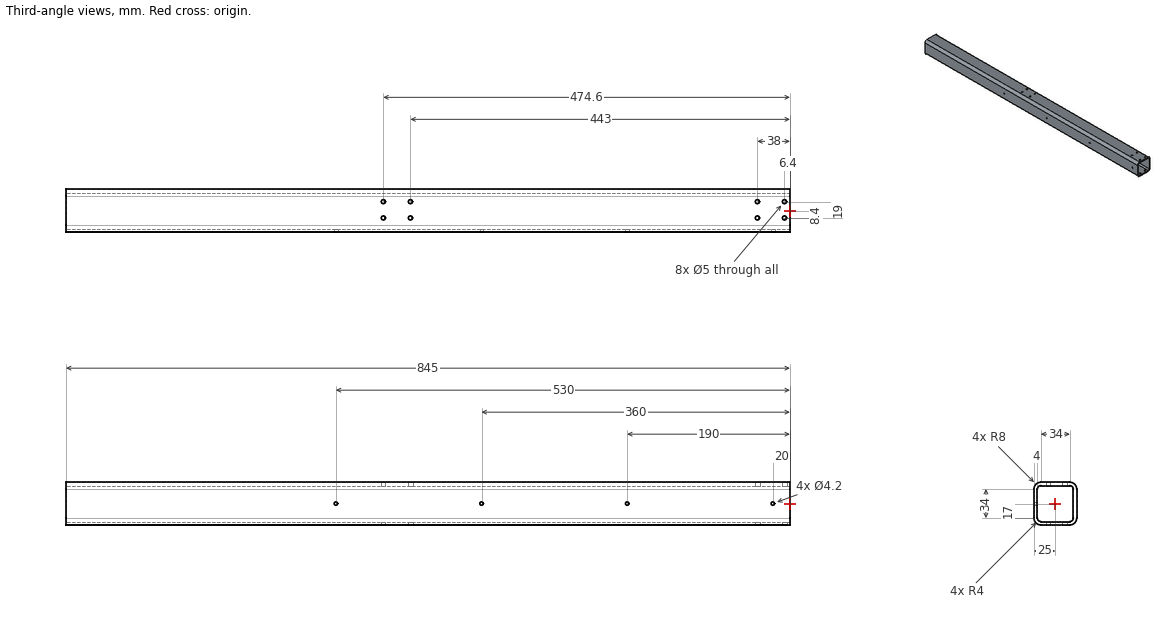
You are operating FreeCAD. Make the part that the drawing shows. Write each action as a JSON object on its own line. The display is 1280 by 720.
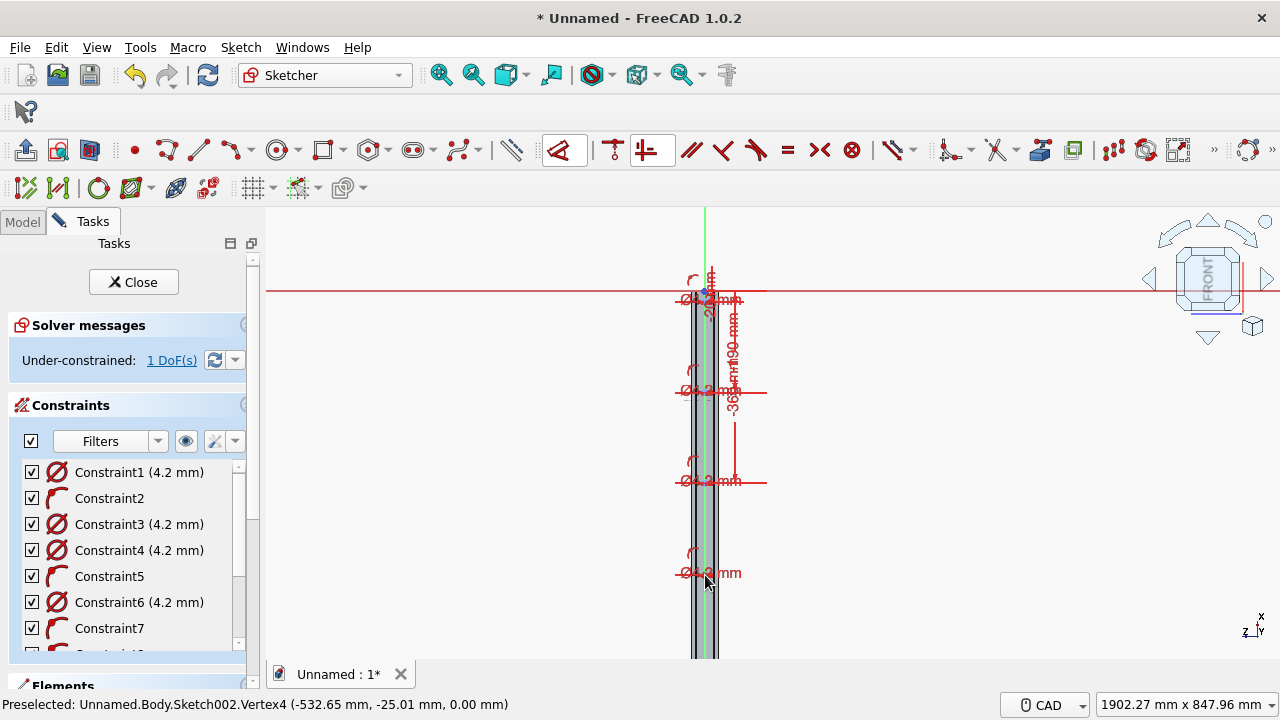
{"action": "left_click", "coordinate": [582, 150]}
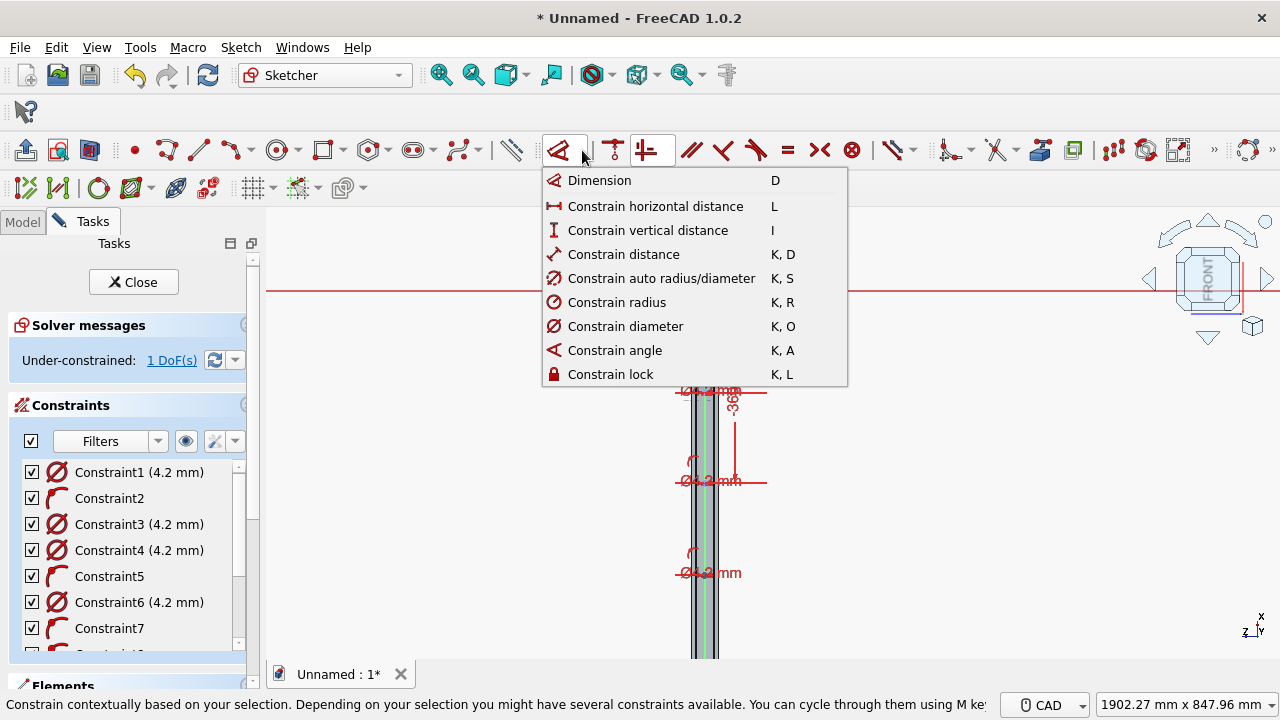
{"action": "left_click", "coordinate": [695, 230]}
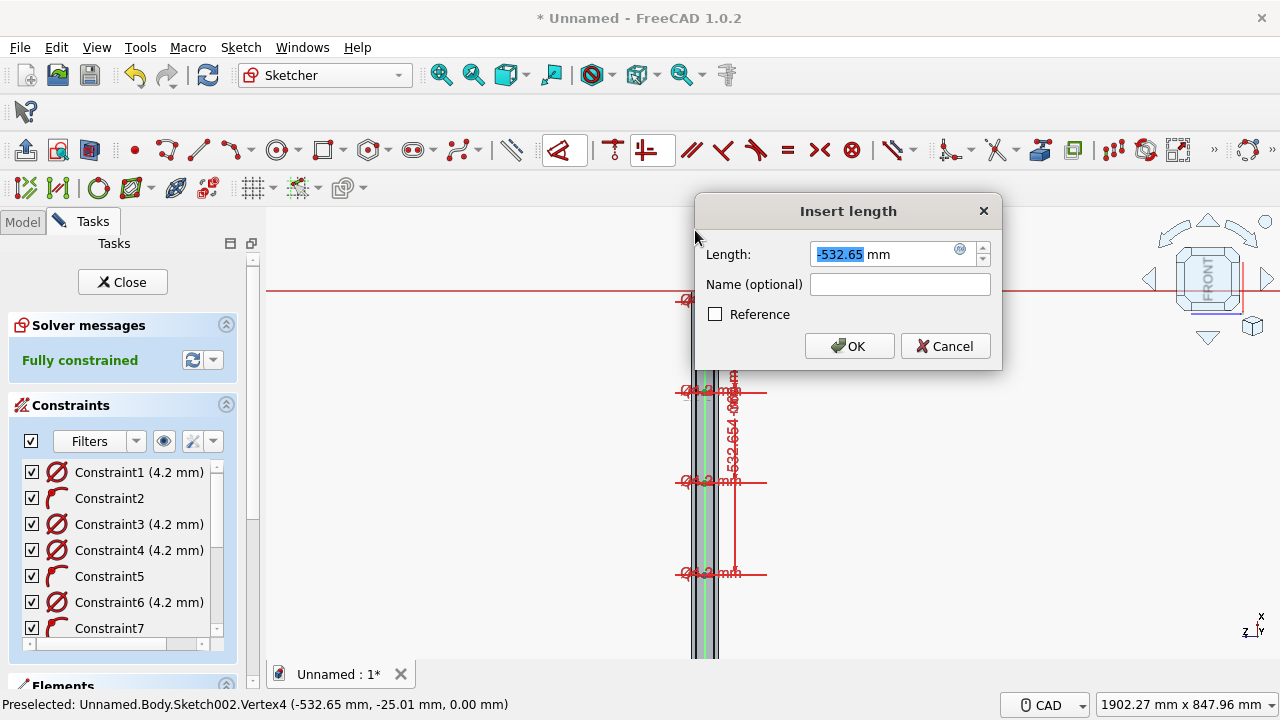
{"action": "type", "text": "-530"}
{"action": "key", "text": "Return"}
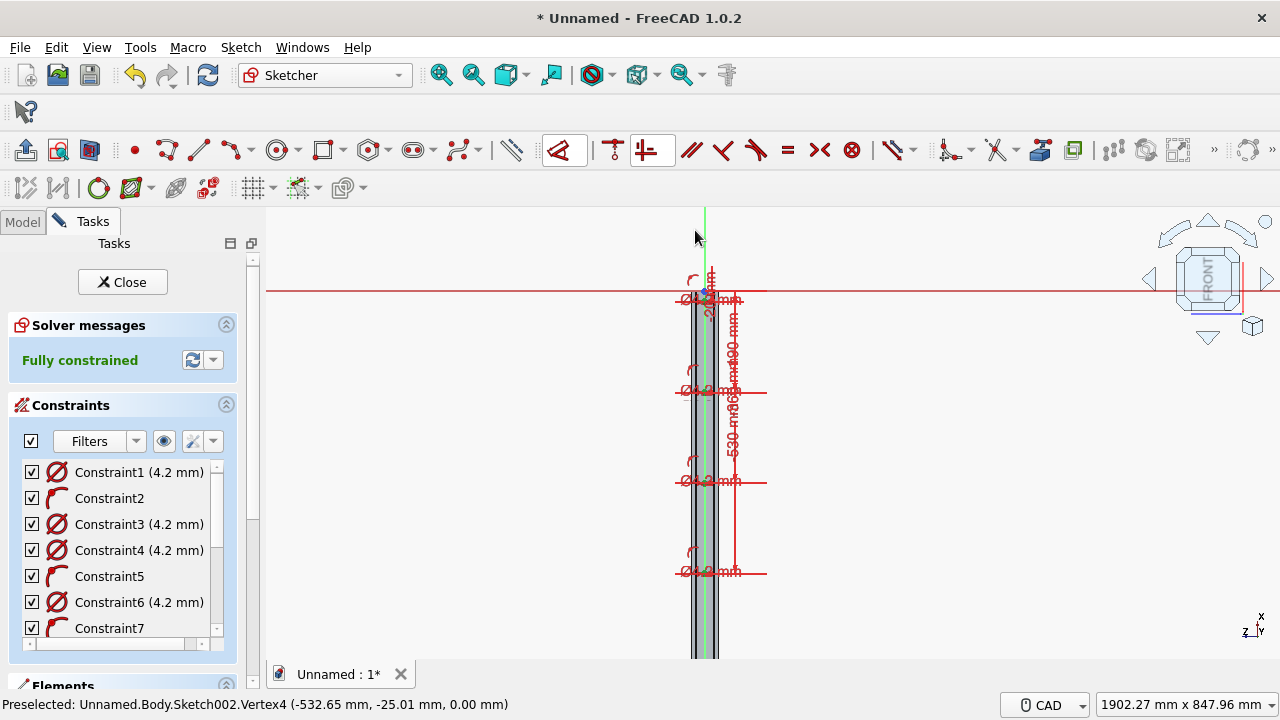
{"action": "left_click", "coordinate": [123, 282]}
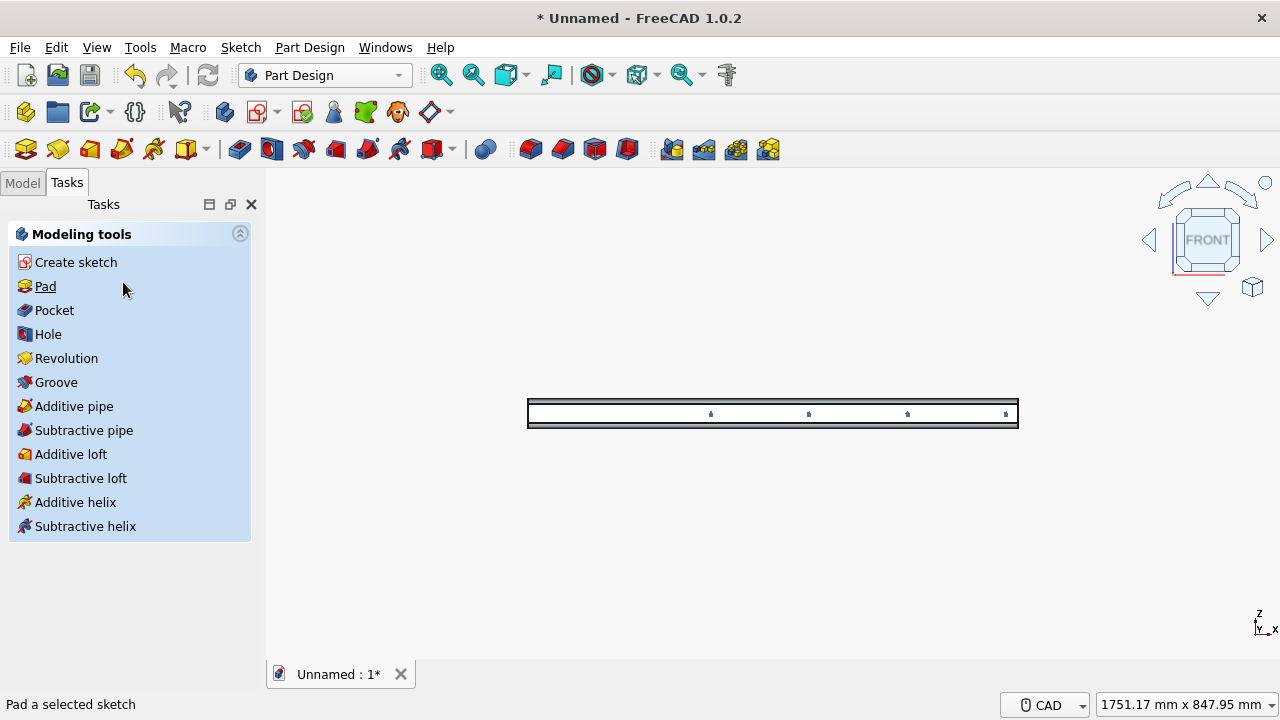
{"action": "left_click", "coordinate": [240, 150]}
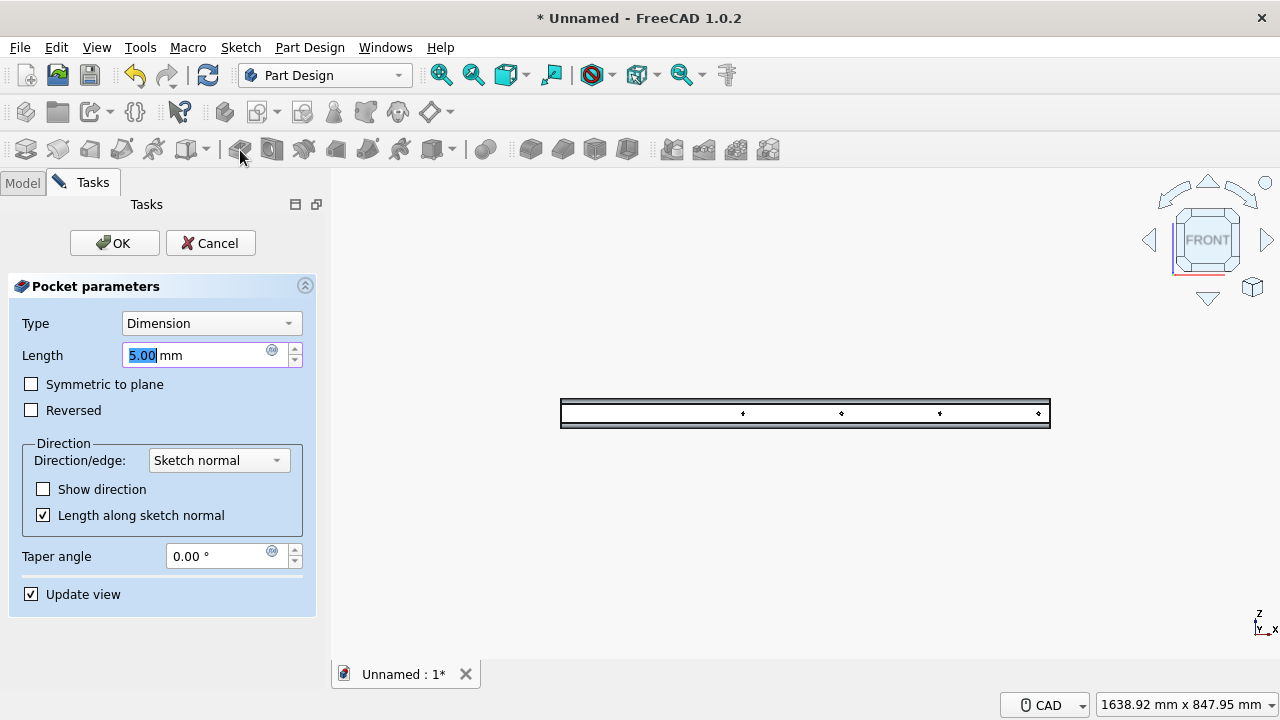
{"action": "type", "text": "4"}
{"action": "key", "text": "Tab"}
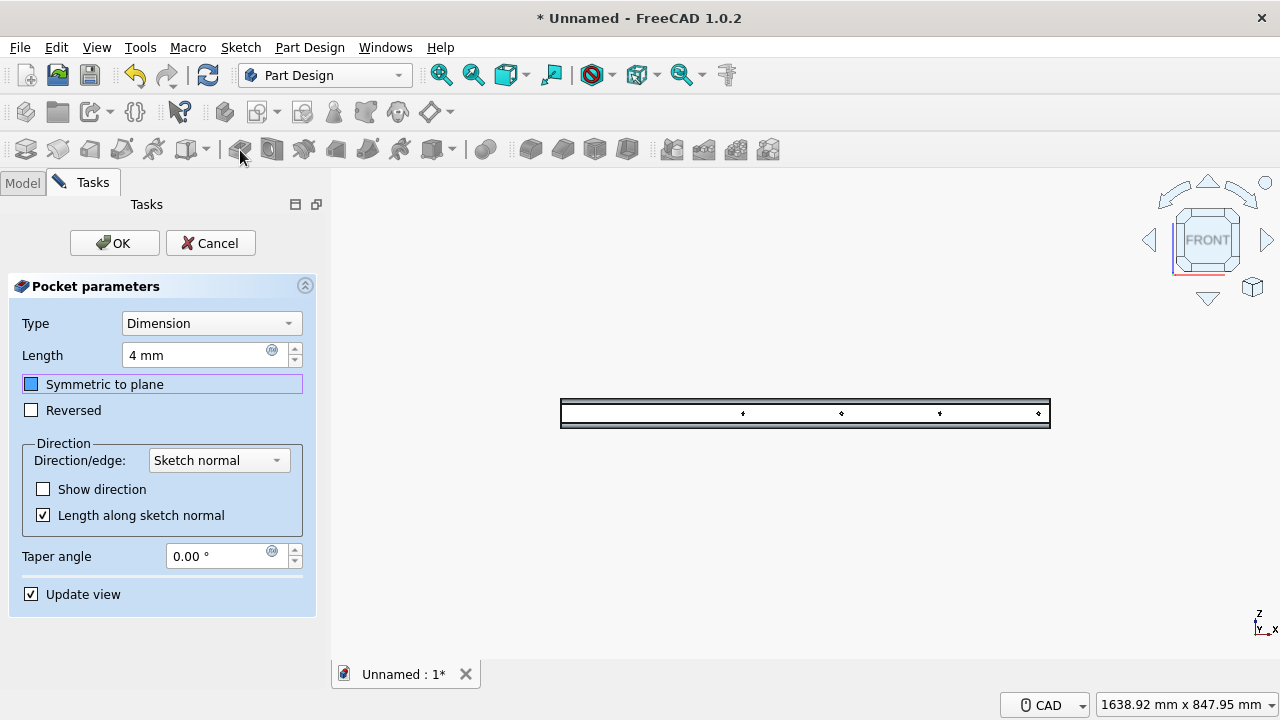
{"action": "left_click", "coordinate": [115, 243]}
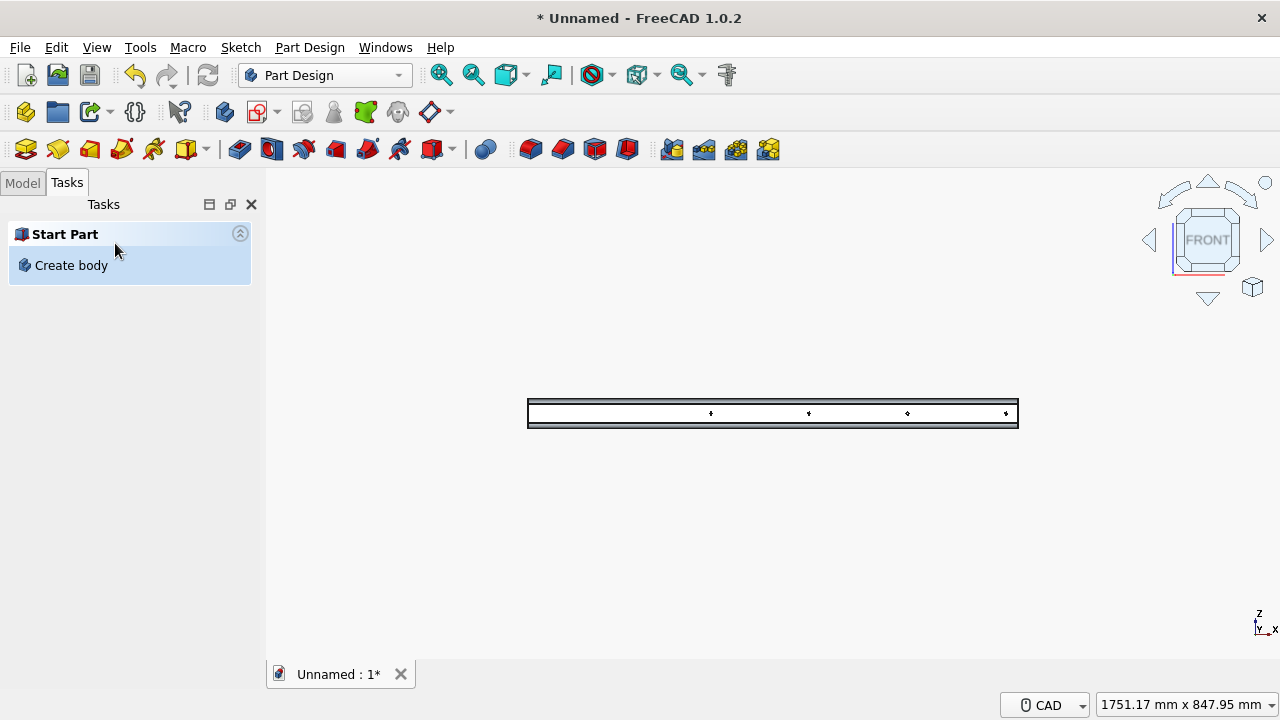
{"action": "key", "text": "0"}